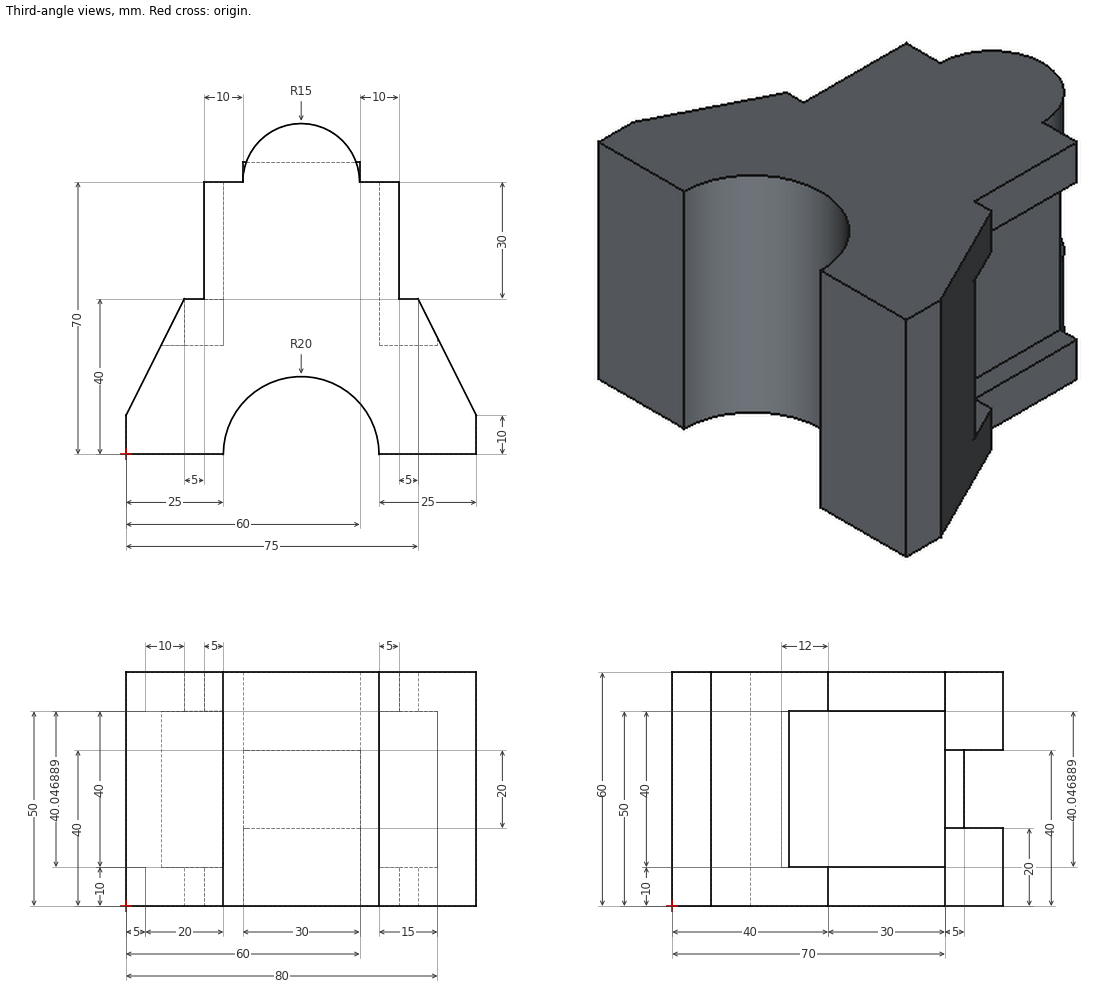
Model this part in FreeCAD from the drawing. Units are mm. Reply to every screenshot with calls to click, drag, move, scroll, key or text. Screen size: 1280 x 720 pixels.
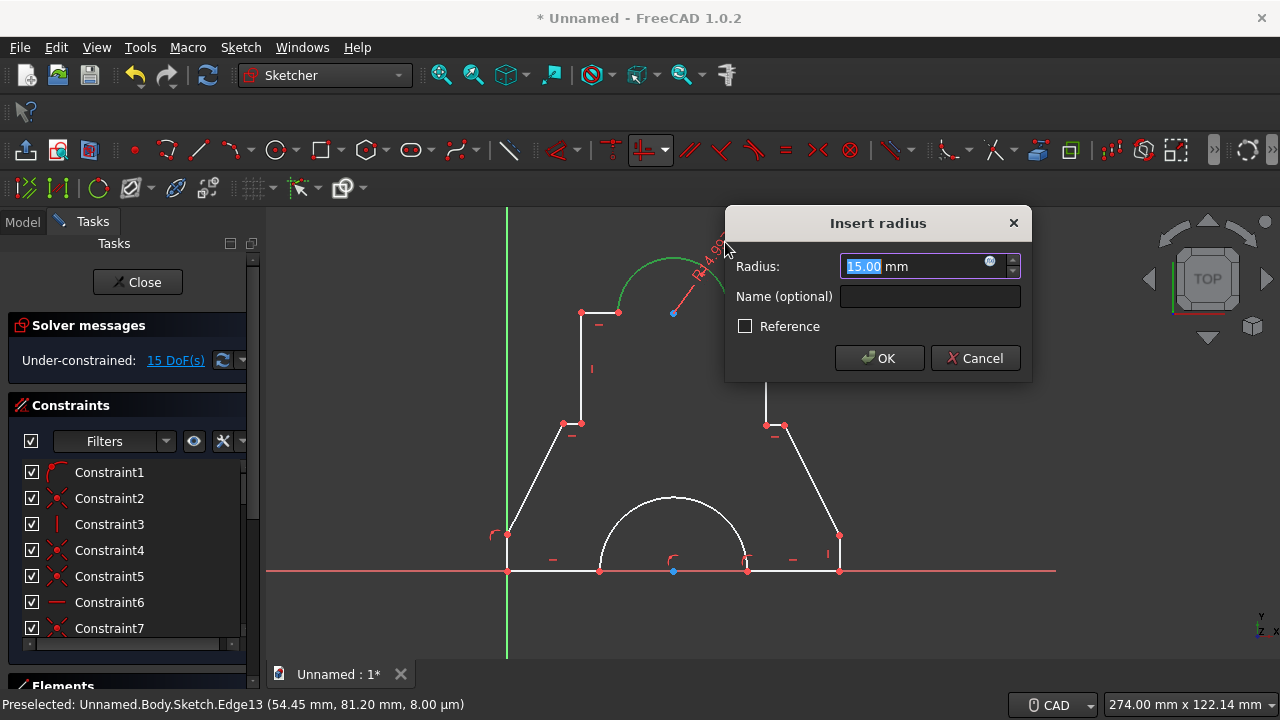
text(15)
key(Return)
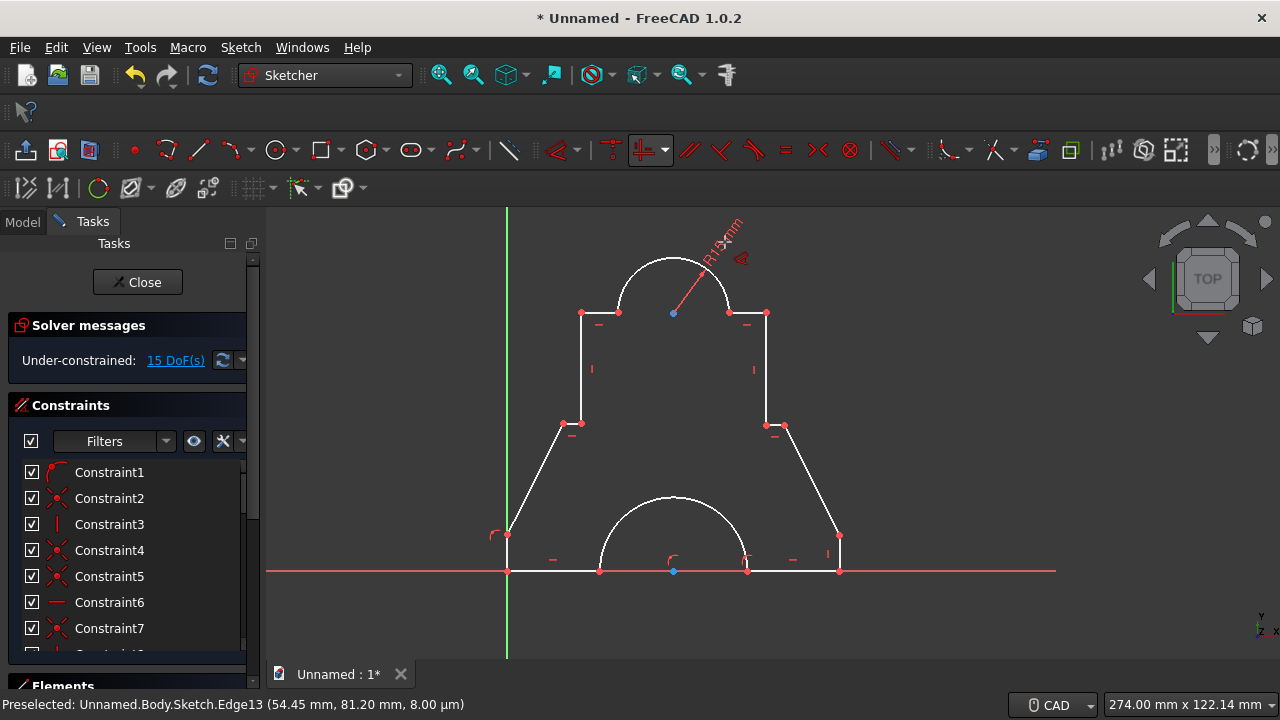
click(717, 511)
click(736, 485)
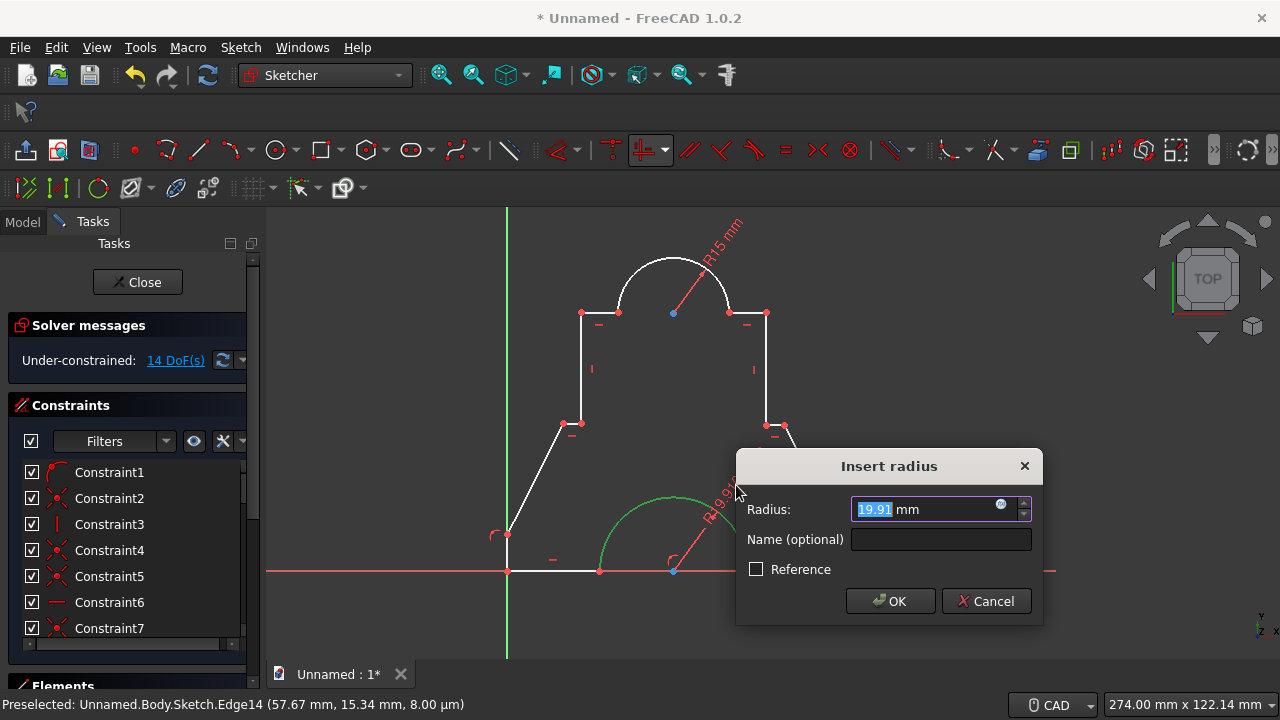
text(20)
key(Return)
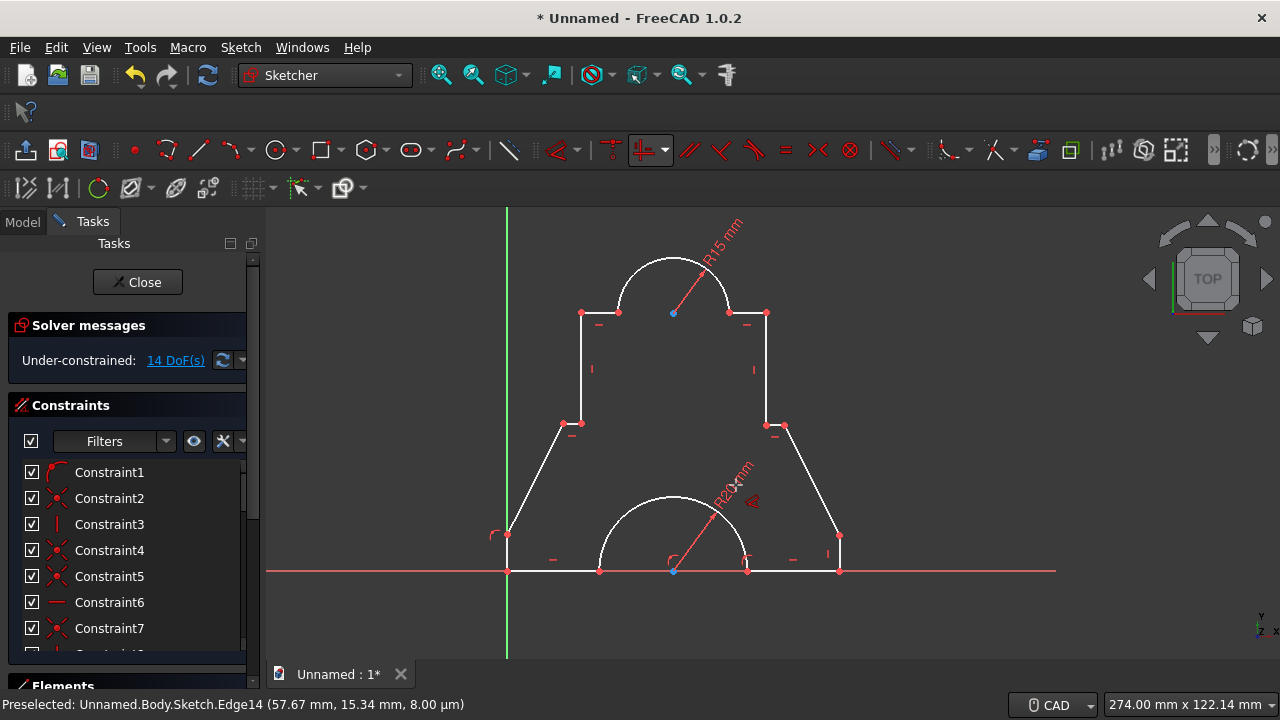
scroll(775, 425, up, 4)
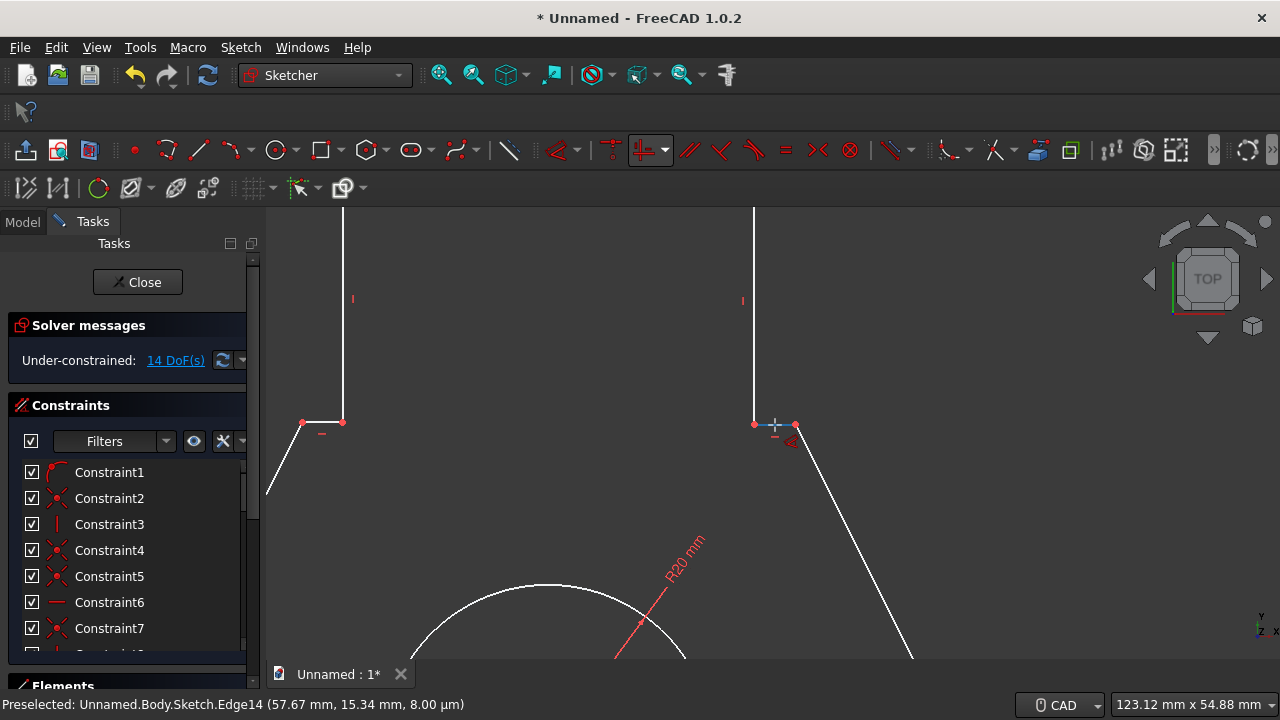
click(775, 425)
click(775, 459)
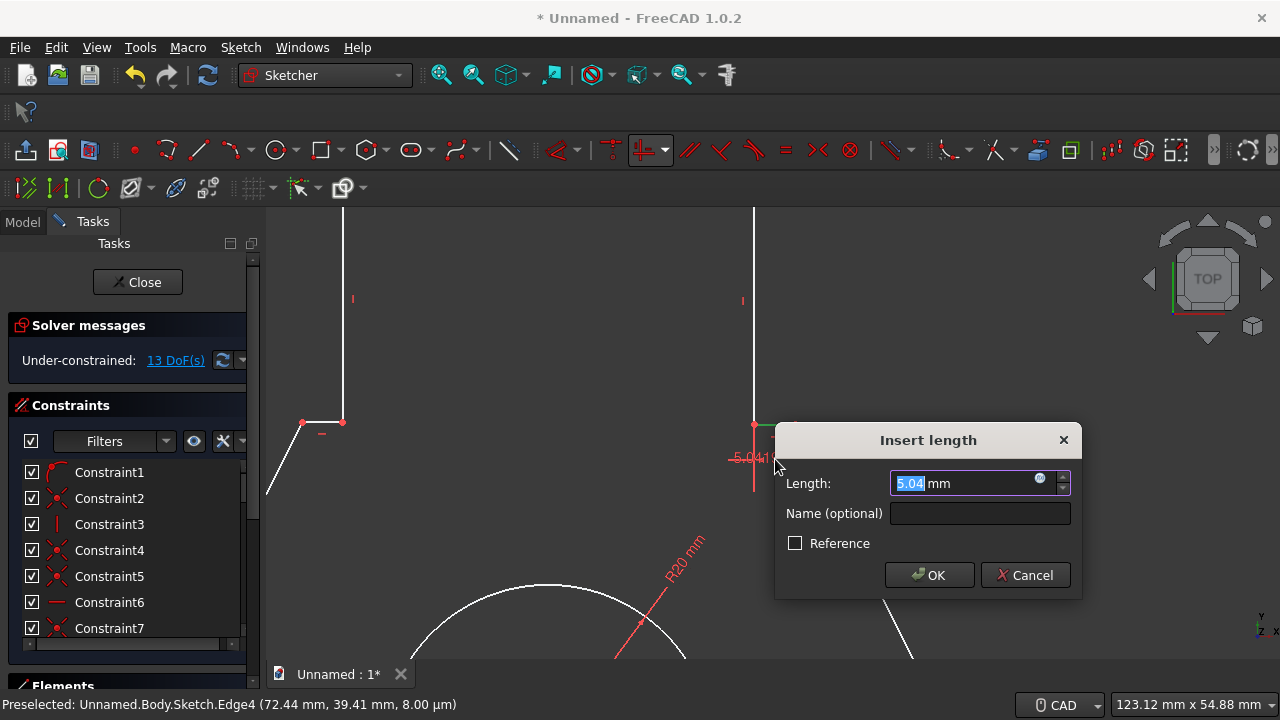
text(5)
key(Return)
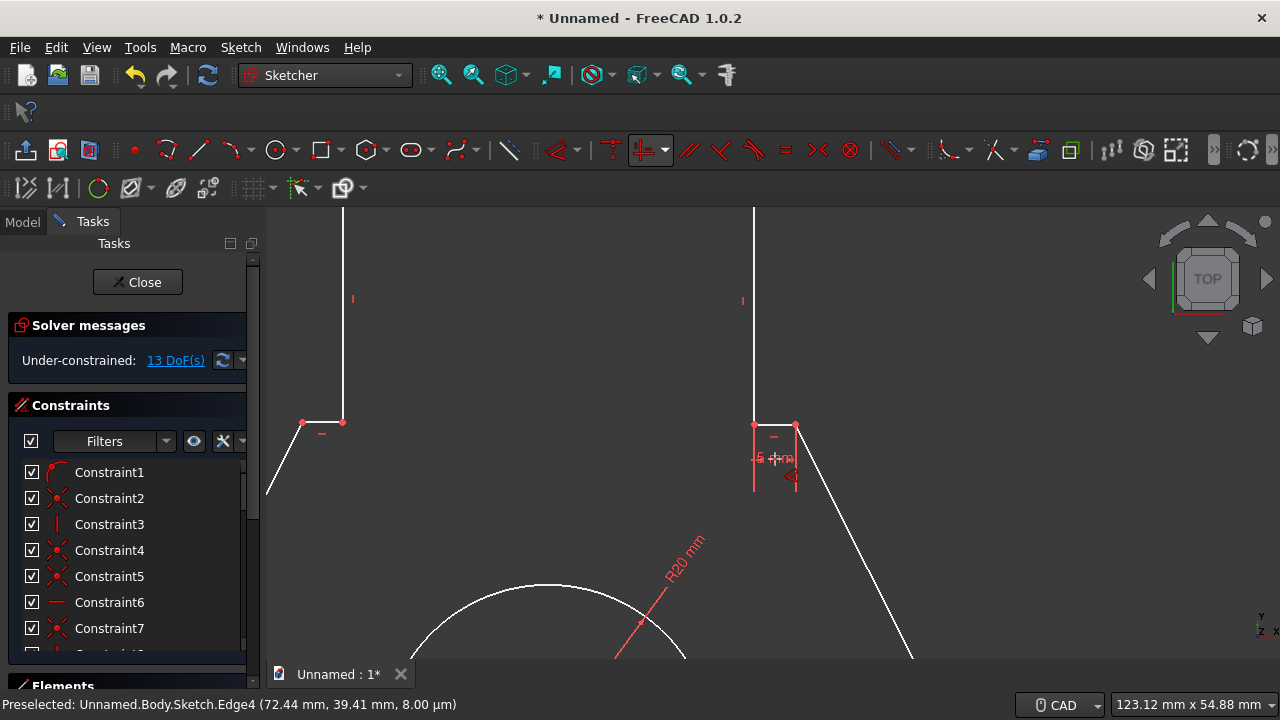
click(331, 422)
click(323, 456)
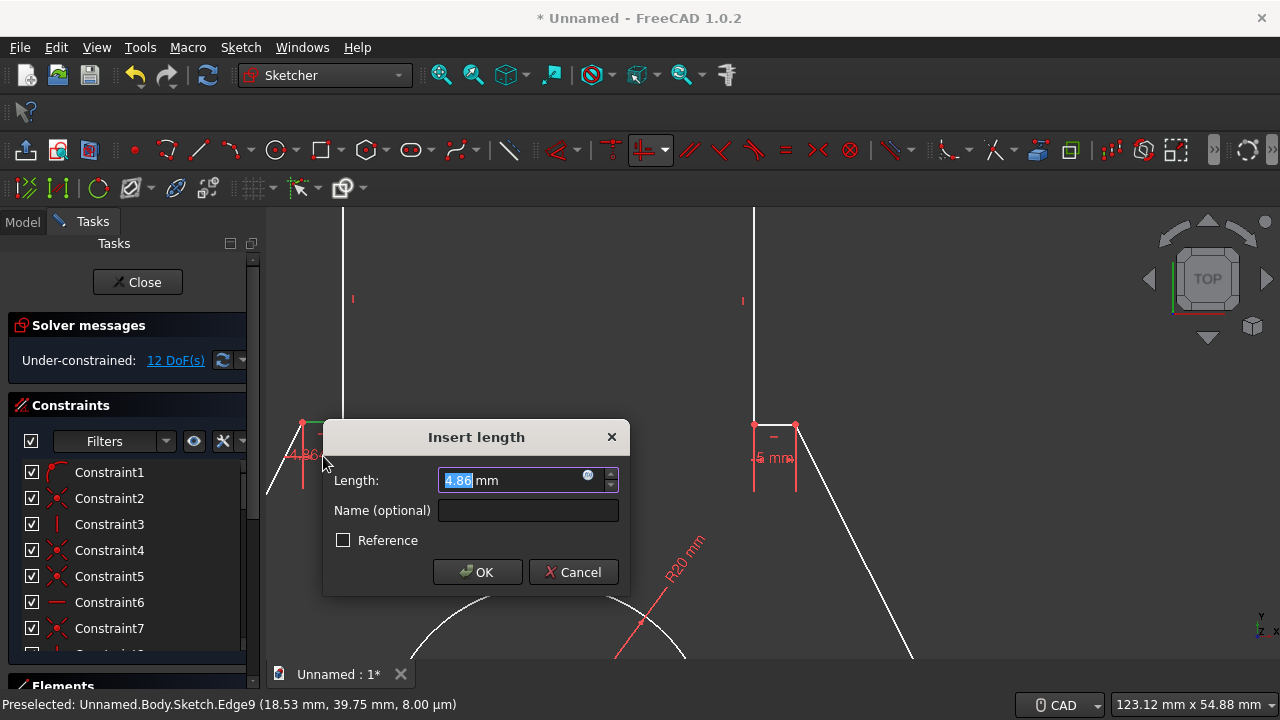
text(5)
key(Return)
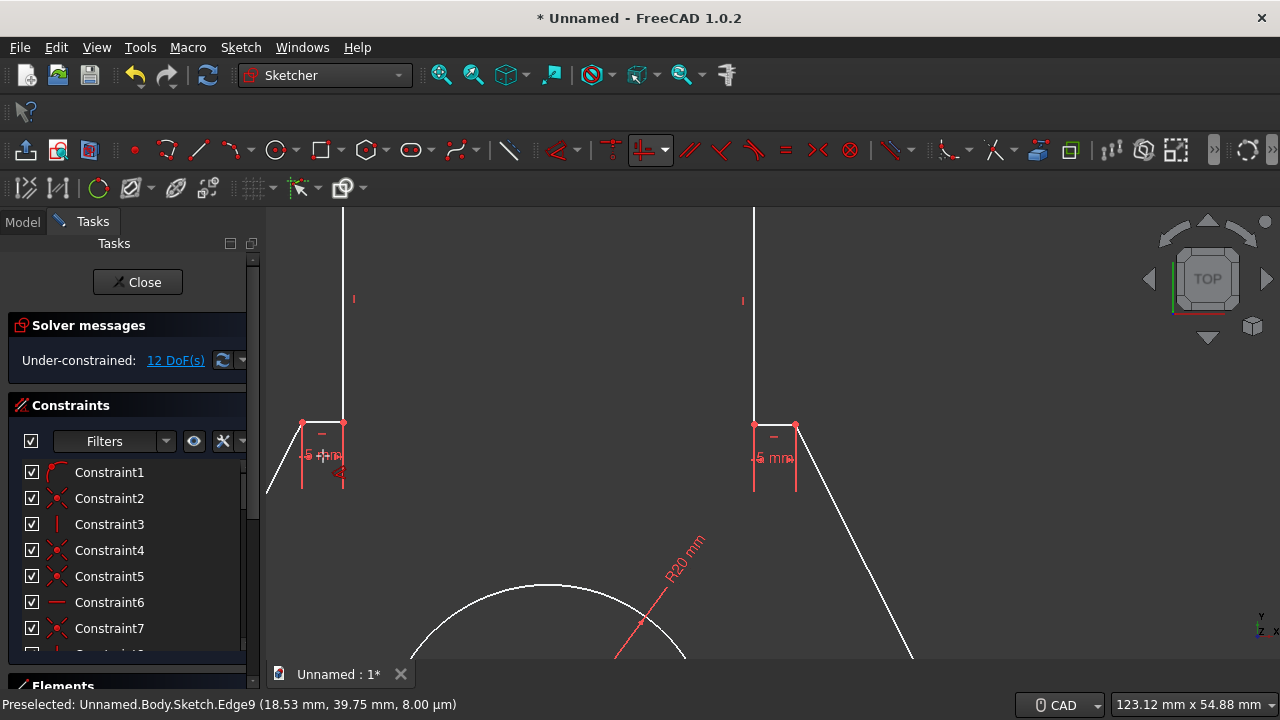
scroll(795, 452, down, 5)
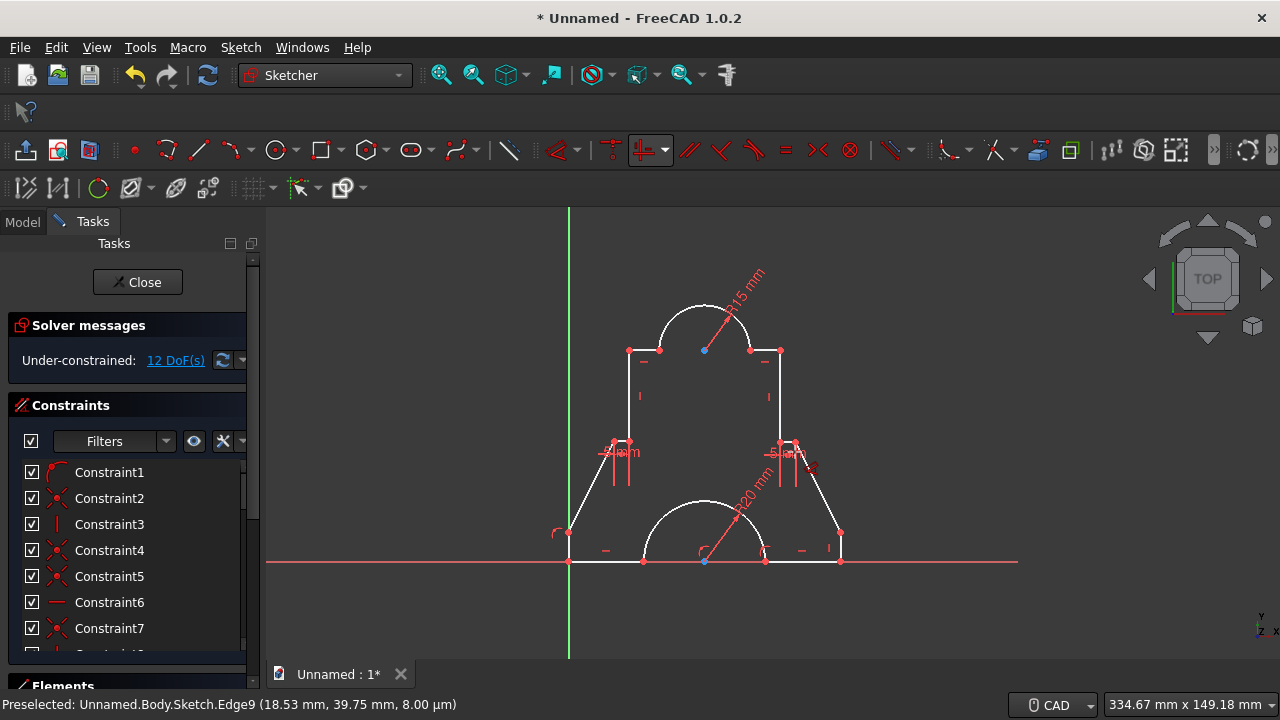
click(788, 562)
click(803, 596)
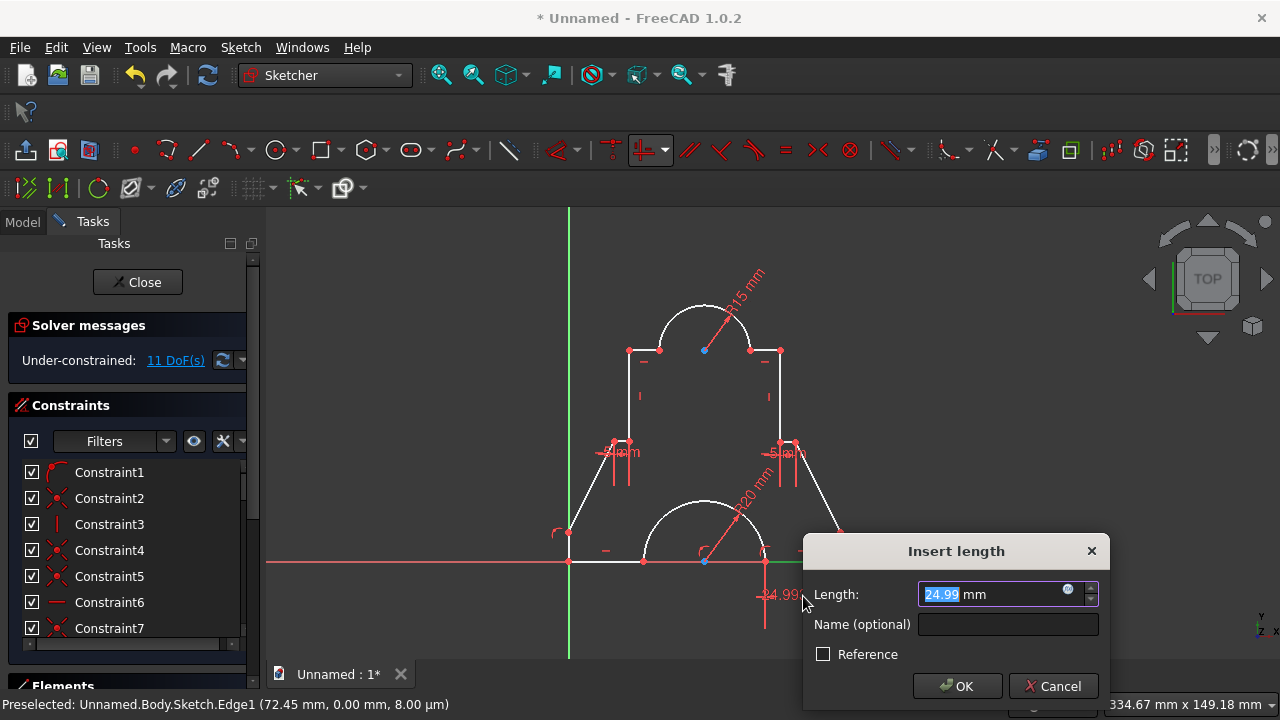
text(25)
key(Return)